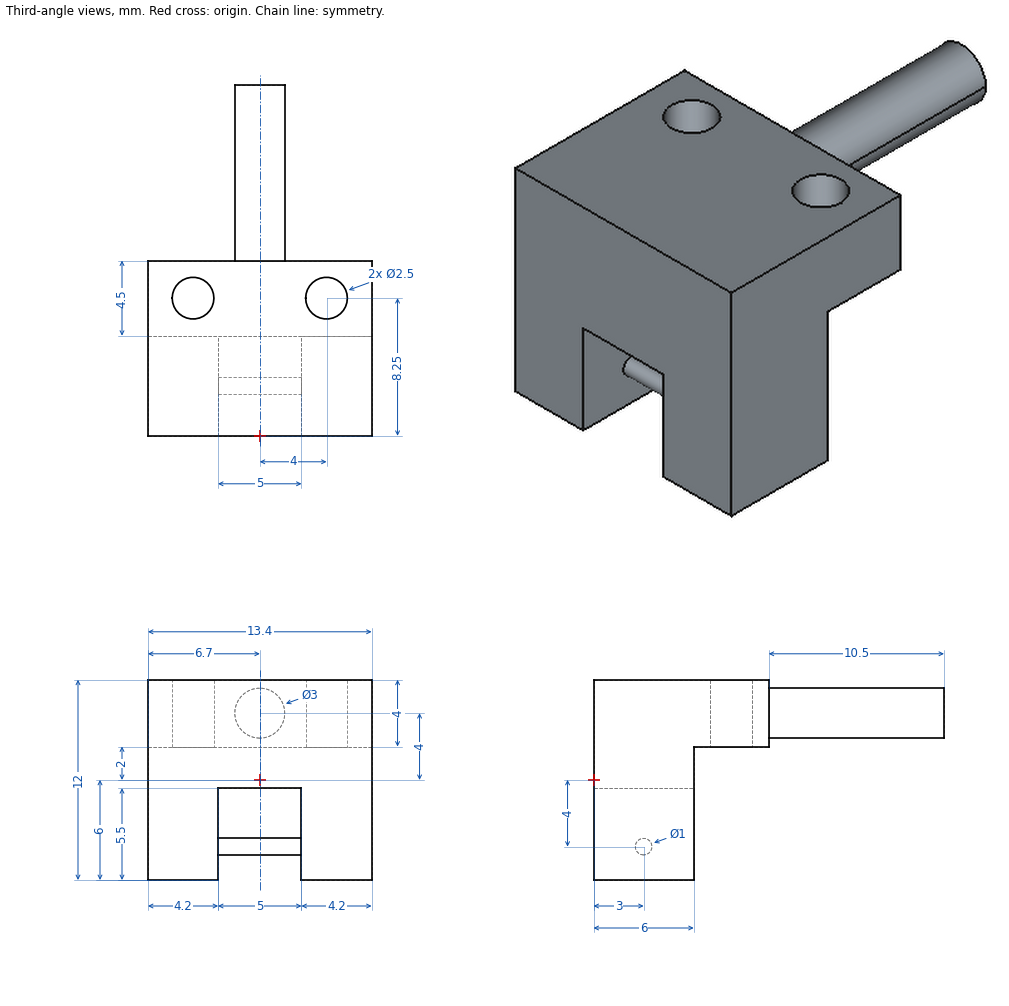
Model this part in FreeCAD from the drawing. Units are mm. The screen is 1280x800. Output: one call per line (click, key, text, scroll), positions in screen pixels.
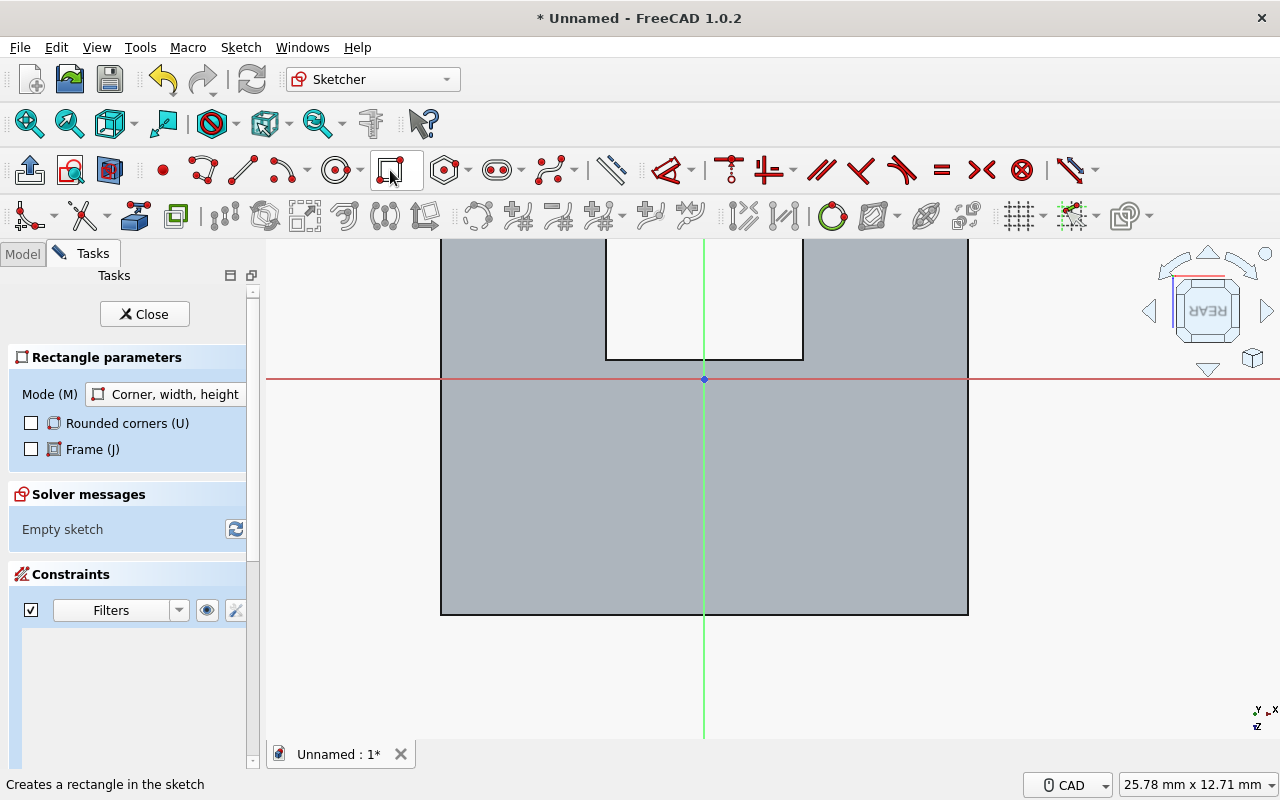
click(441, 458)
move(968, 615)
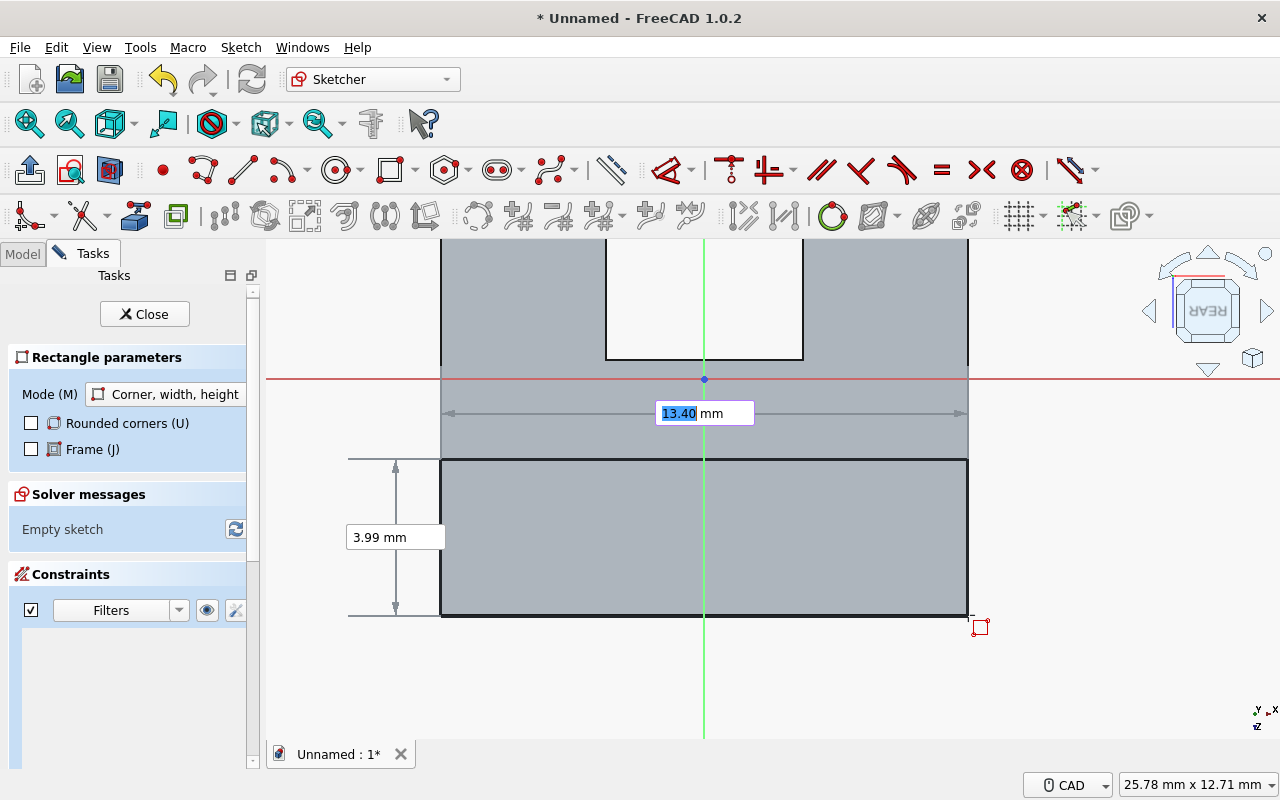
text(13.4)
key(Tab)
text(4)
key(Return)
key(Escape)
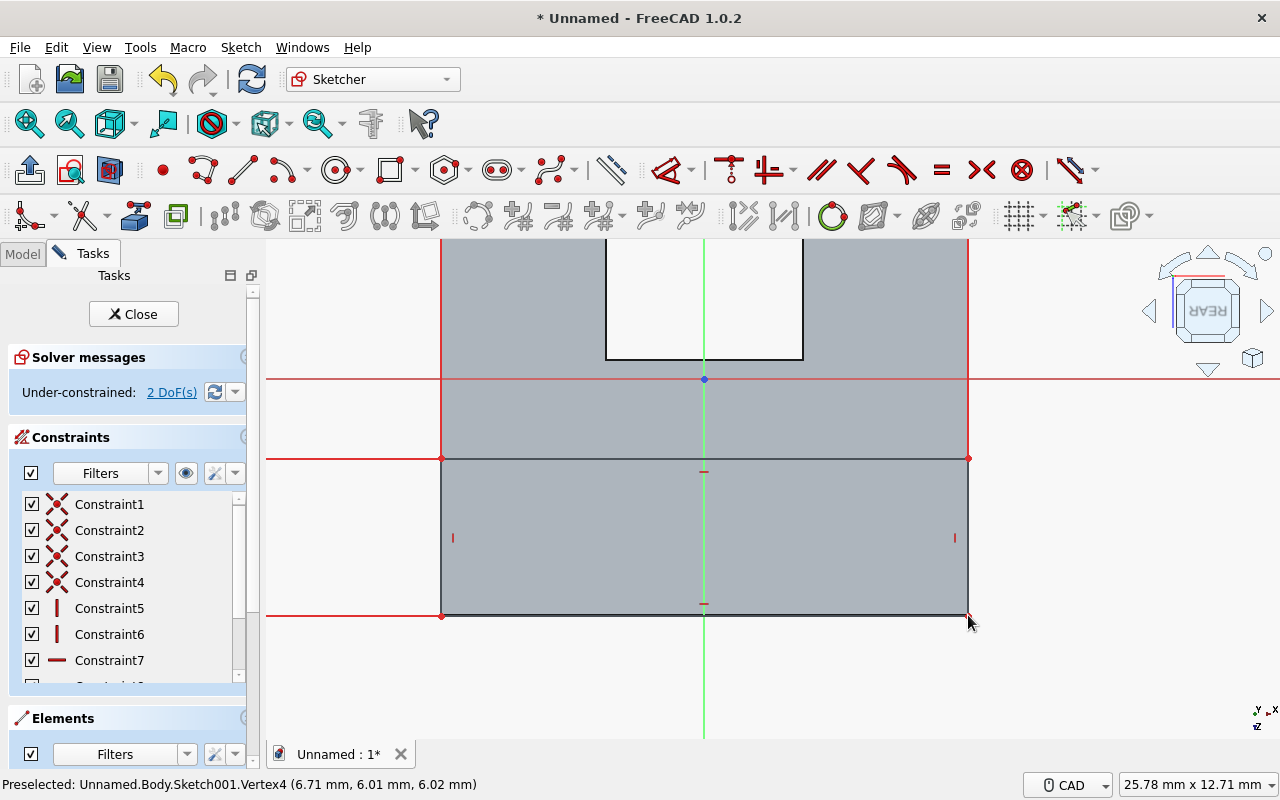
click(666, 170)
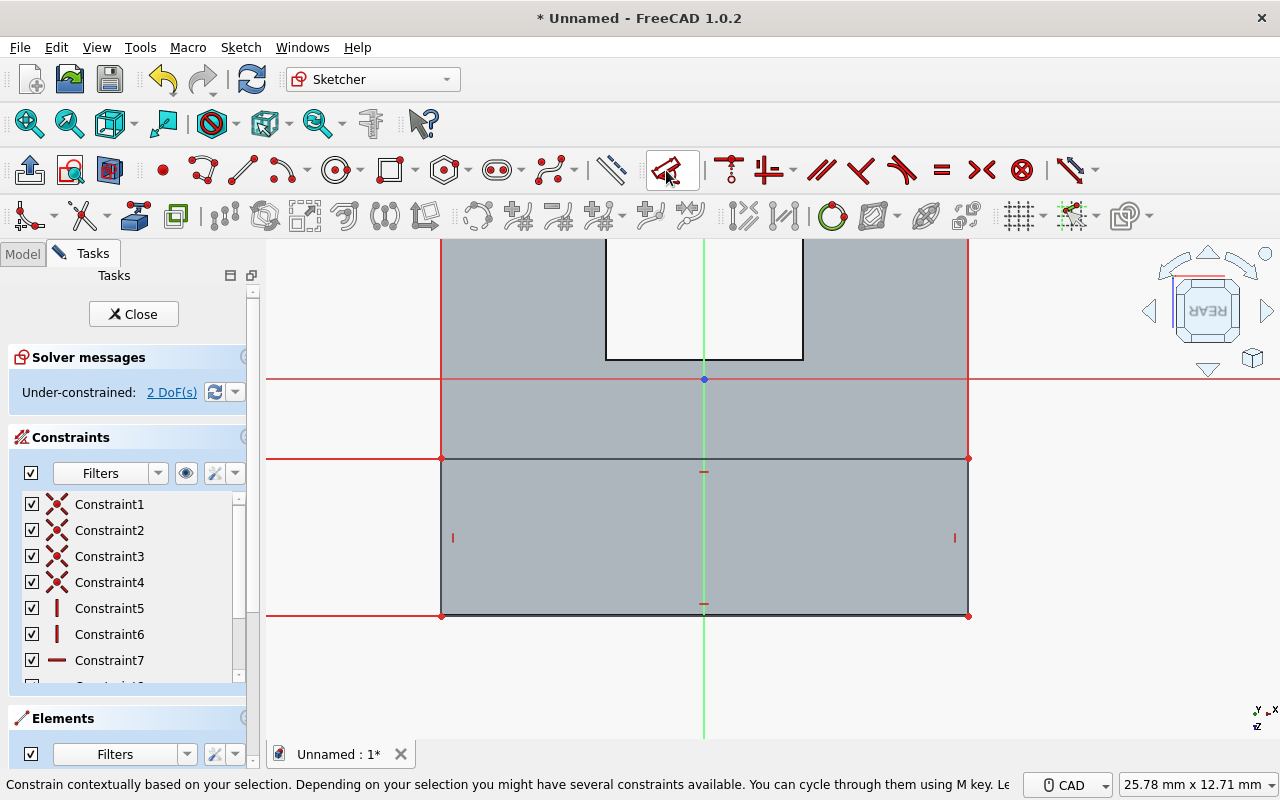
click(441, 459)
click(407, 419)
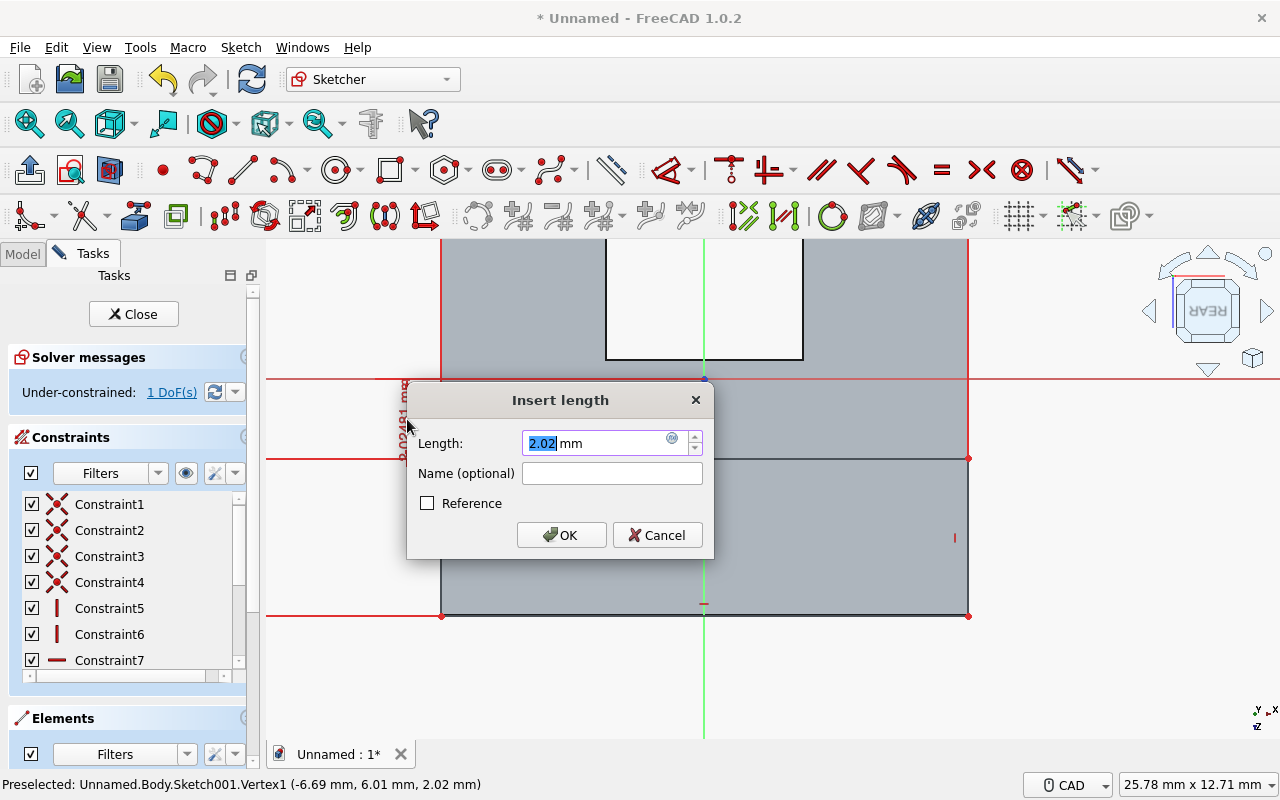
text(2)
key(Return)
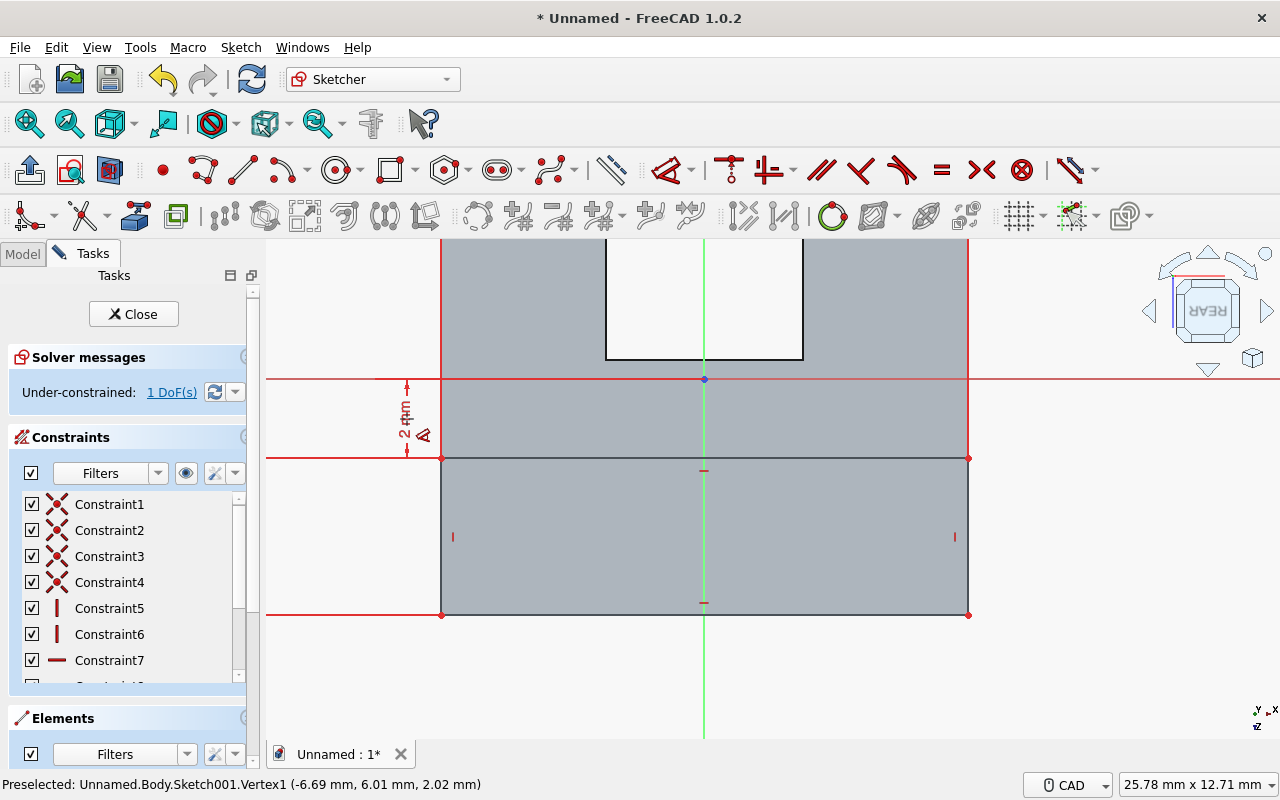
click(441, 458)
click(573, 345)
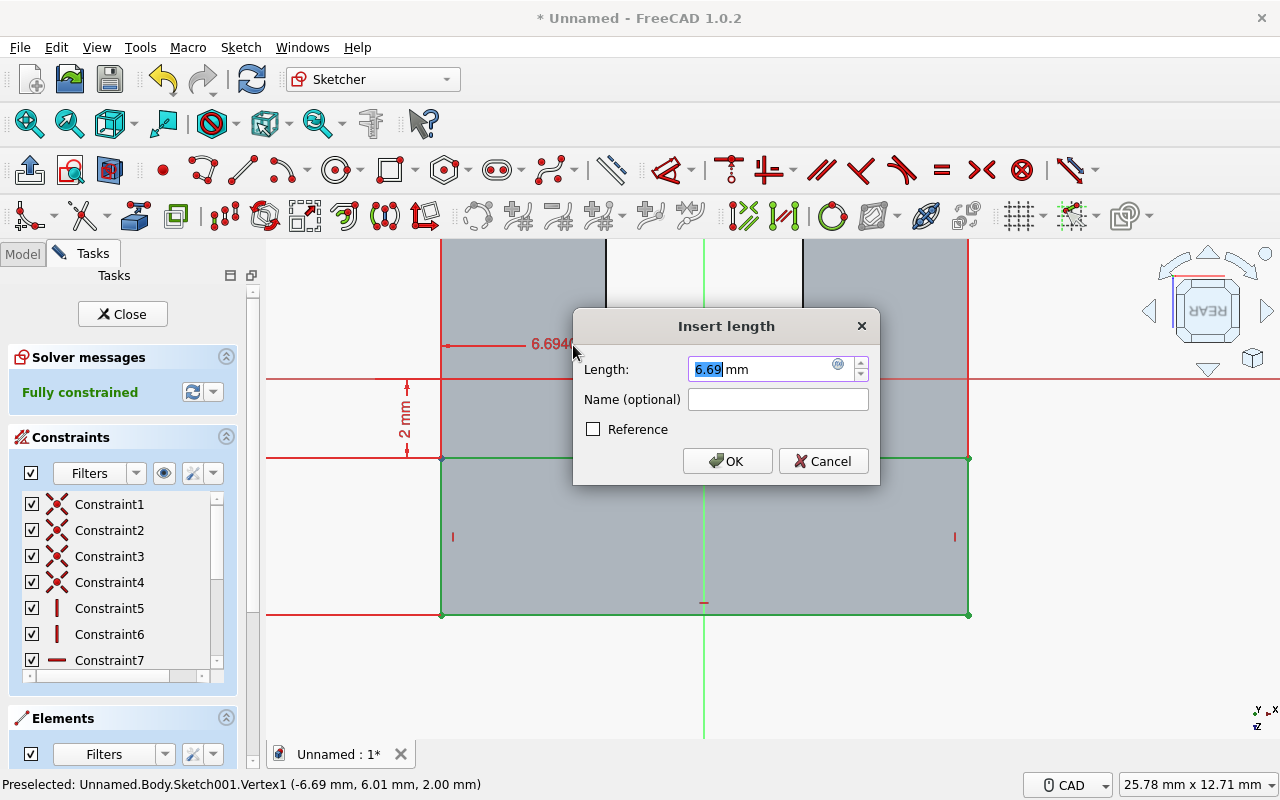
text(6.7)
key(Return)
key(Escape)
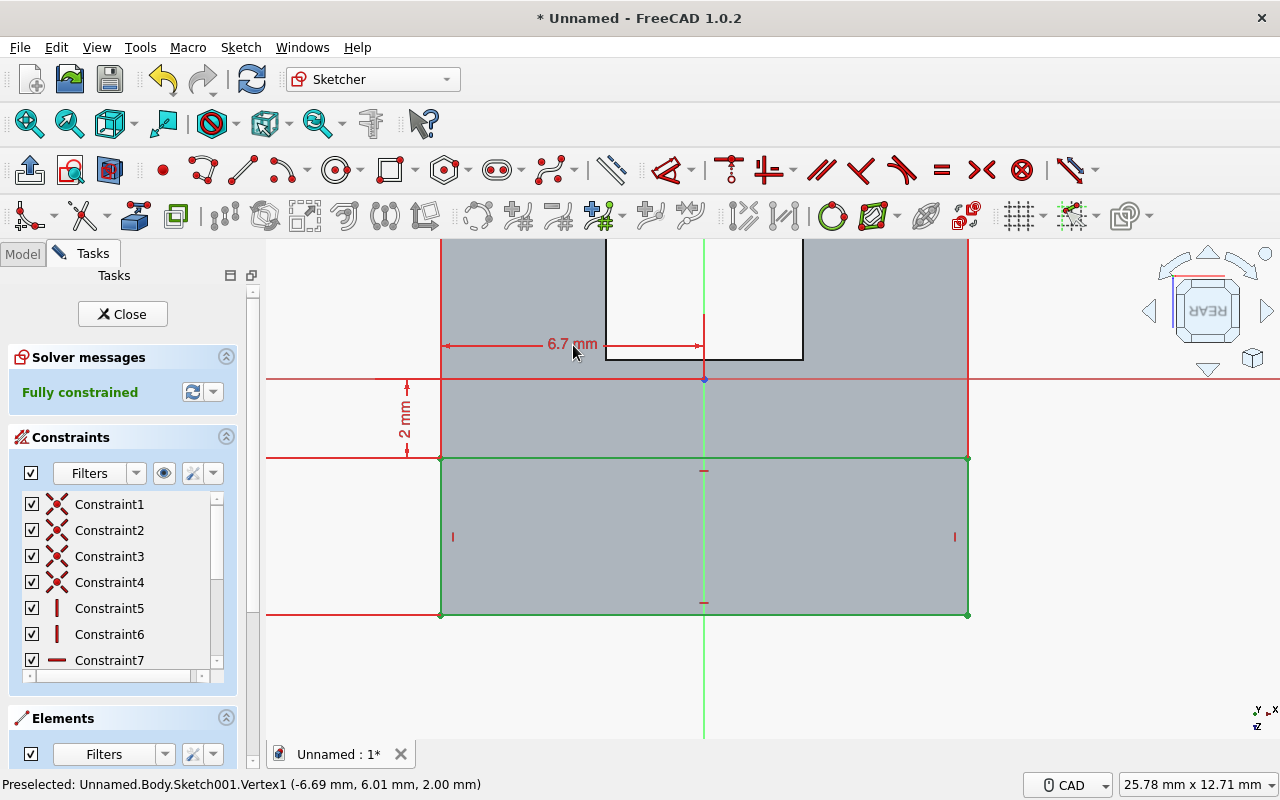
click(123, 314)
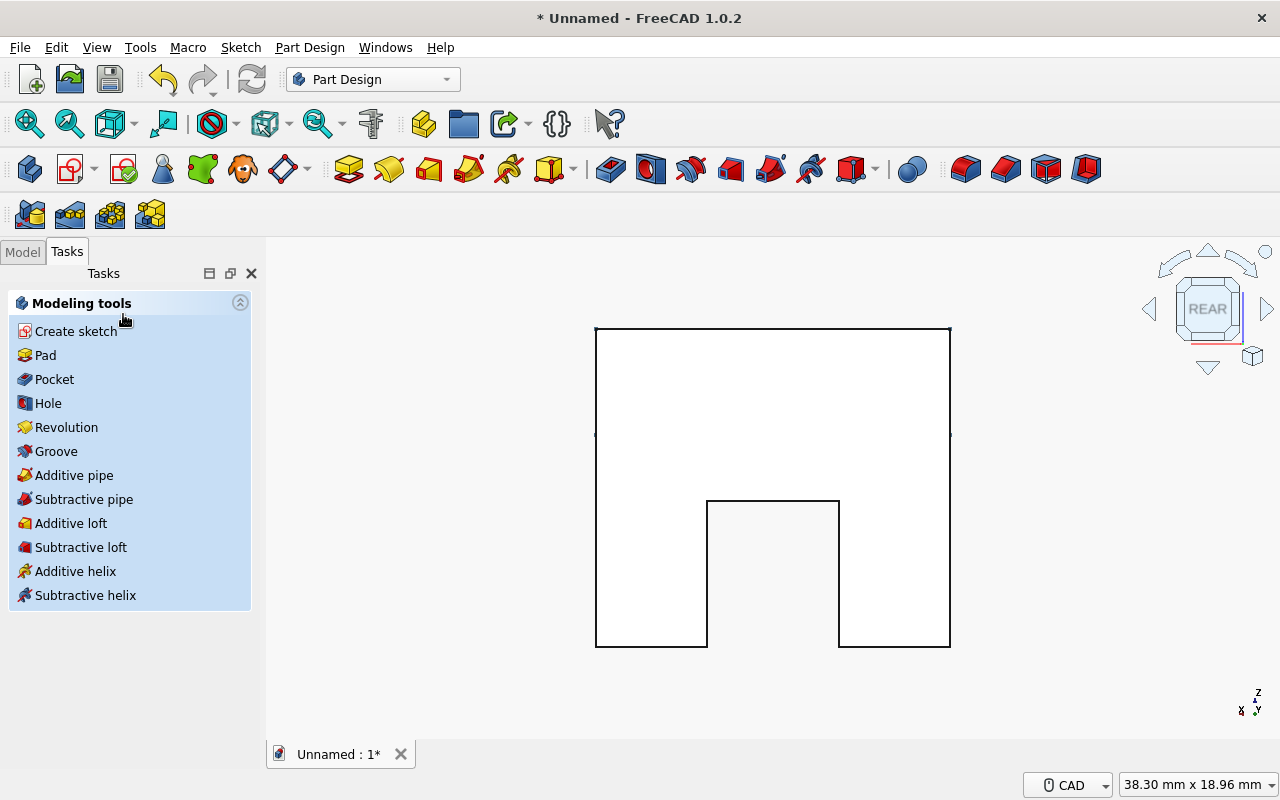
click(350, 170)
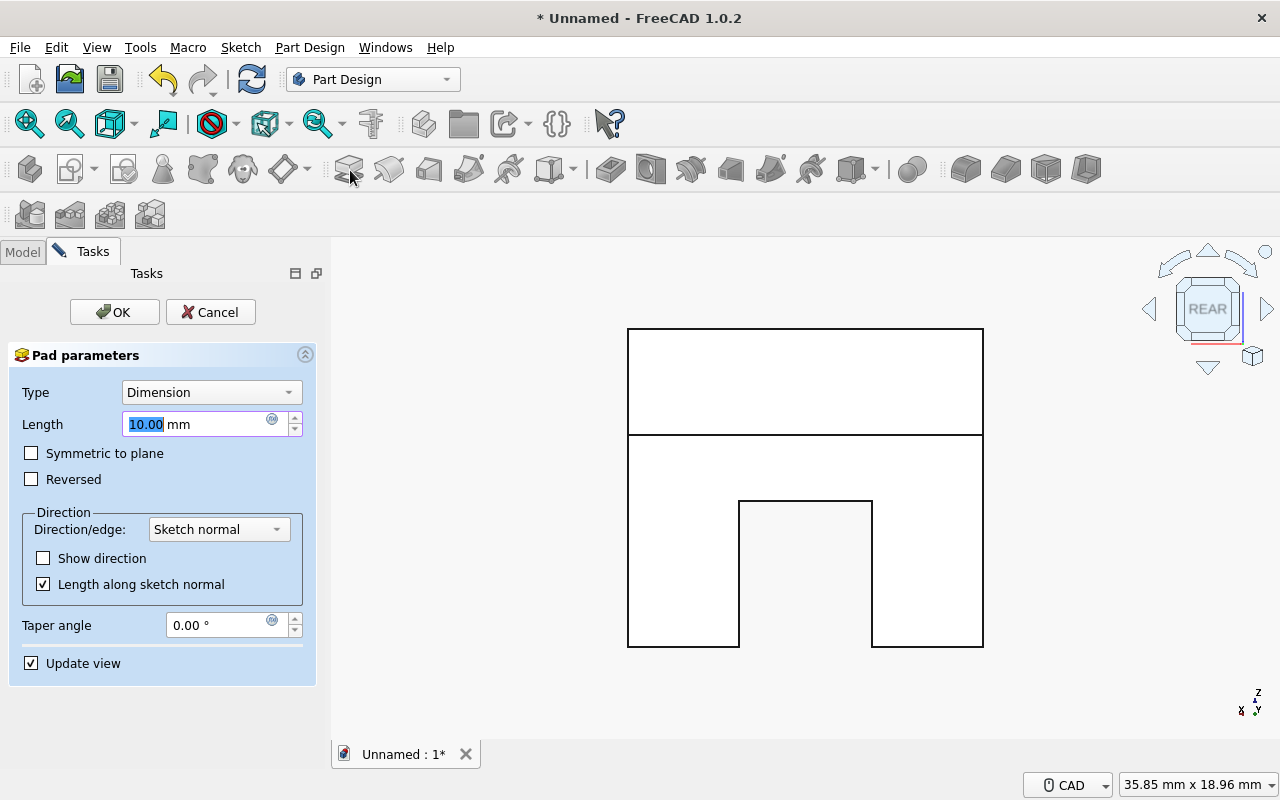
text(4.5)
key(Tab)